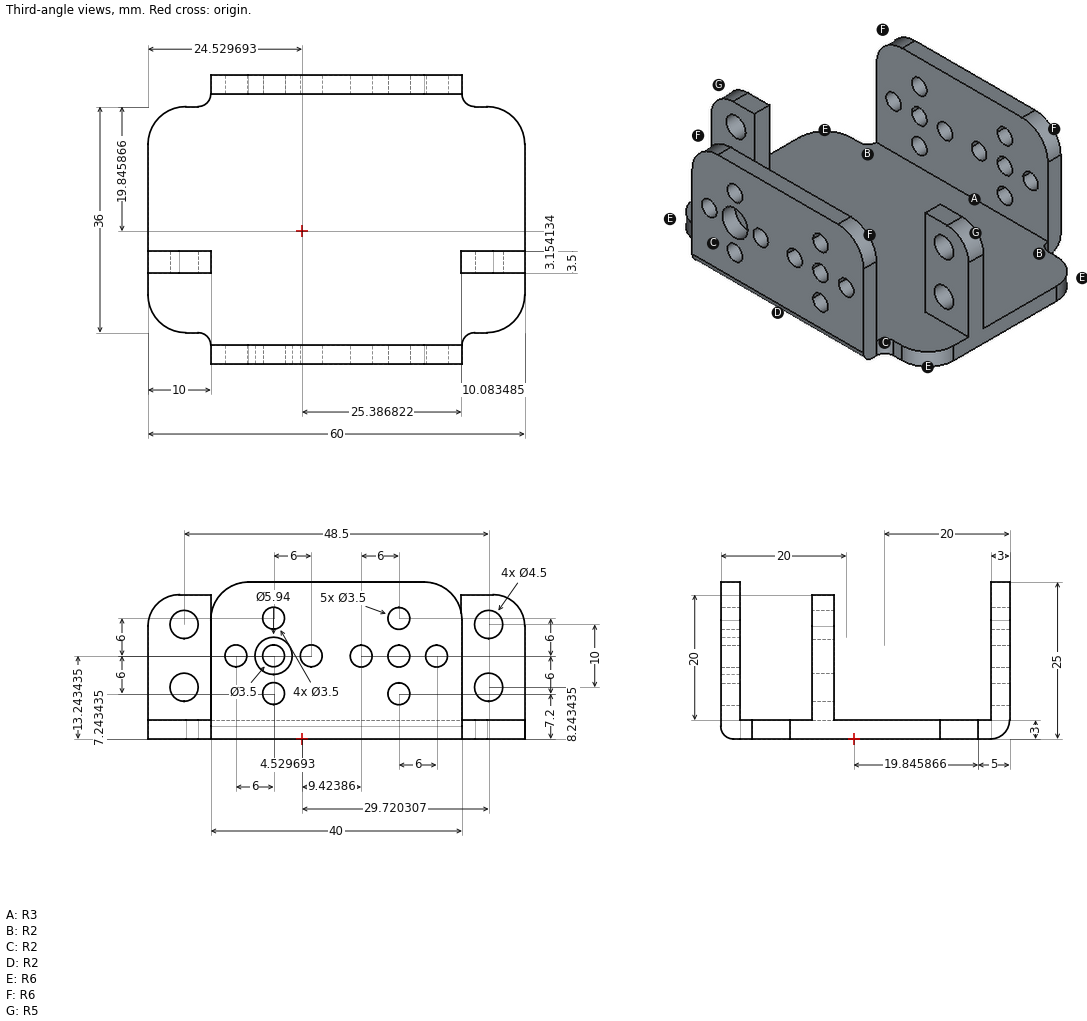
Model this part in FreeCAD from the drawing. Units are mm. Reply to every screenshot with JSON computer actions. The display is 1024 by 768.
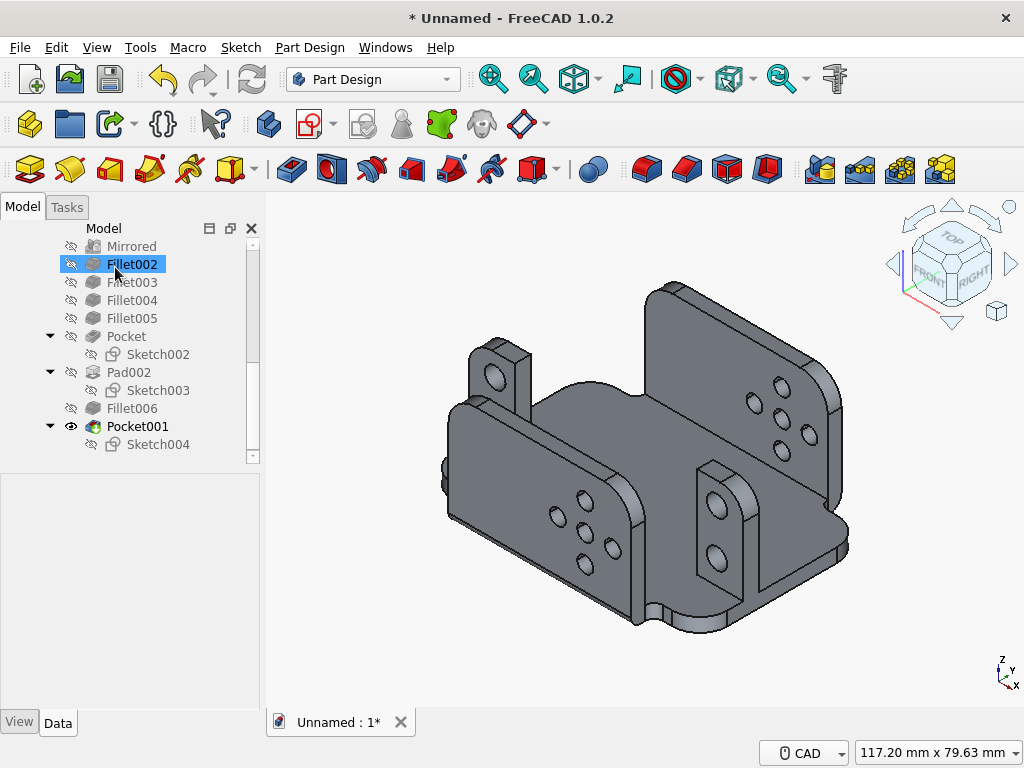
{"action": "left_click", "coordinate": [488, 474]}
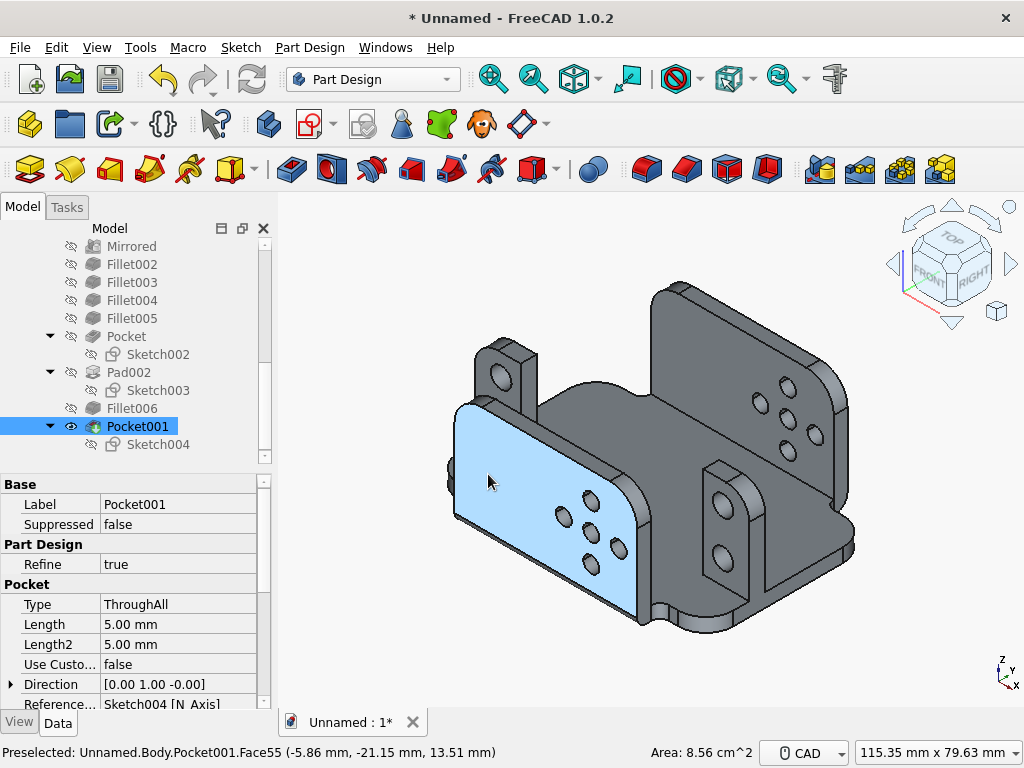
{"action": "left_click", "coordinate": [310, 124]}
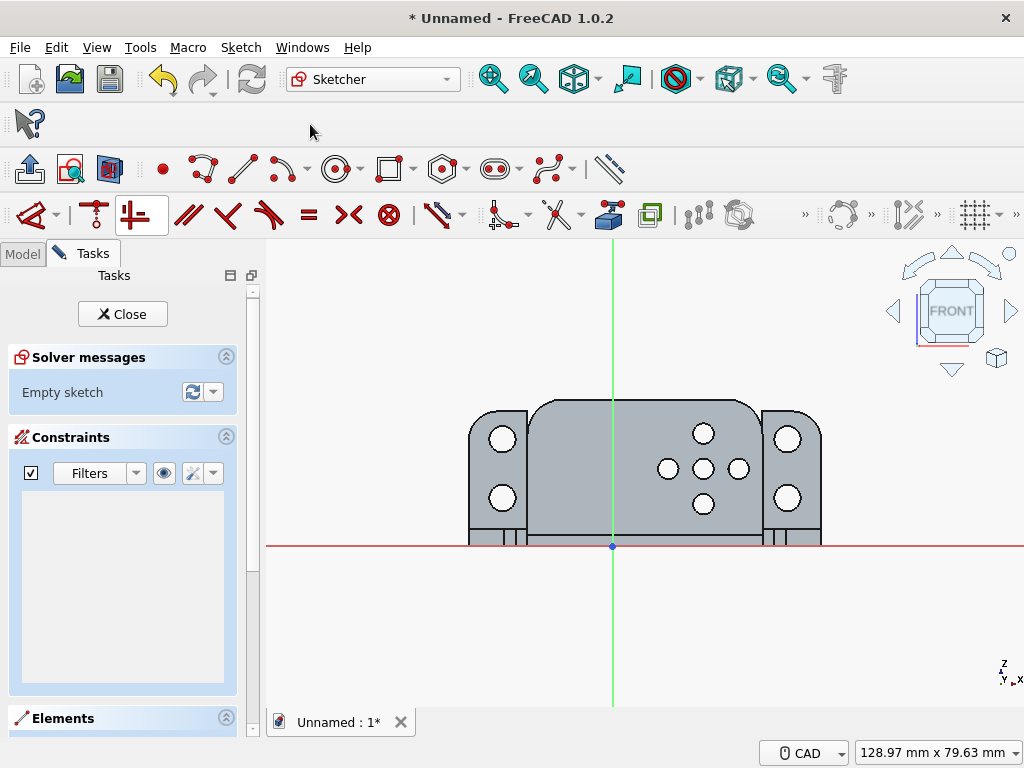
{"action": "scroll", "coordinate": [587, 468], "scroll_direction": "up", "scroll_amount": 11}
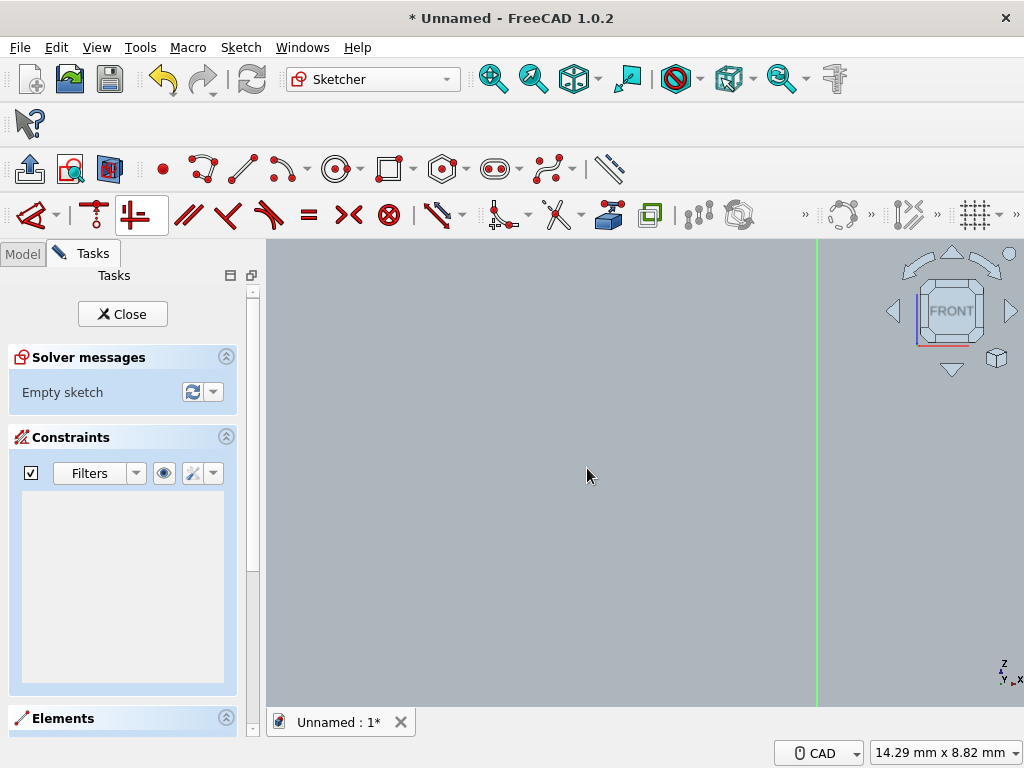
{"action": "left_click", "coordinate": [336, 170]}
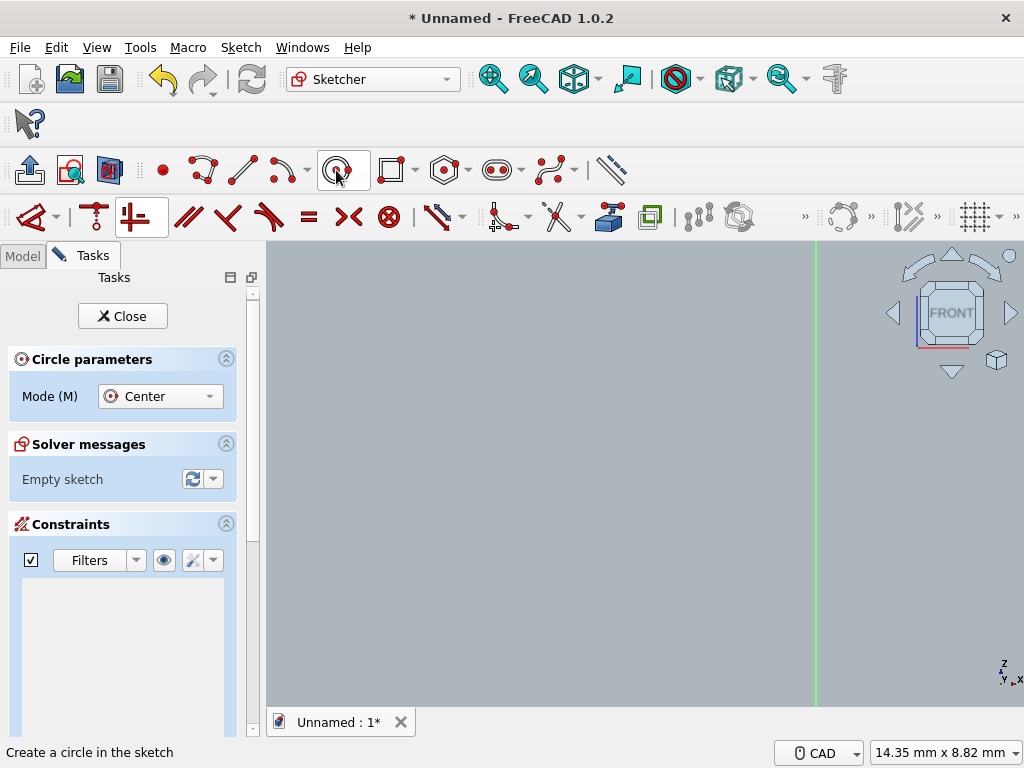
{"action": "left_click", "coordinate": [577, 471]}
{"action": "left_click", "coordinate": [688, 360]}
{"action": "key", "text": "Escape"}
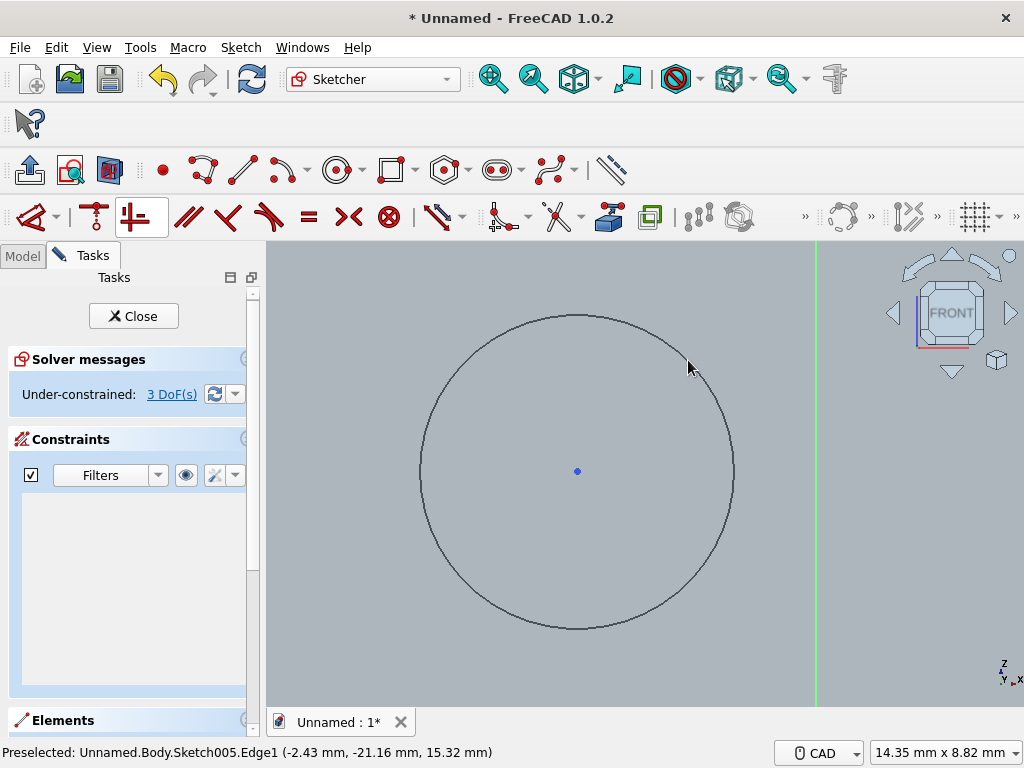
{"action": "left_click", "coordinate": [32, 218]}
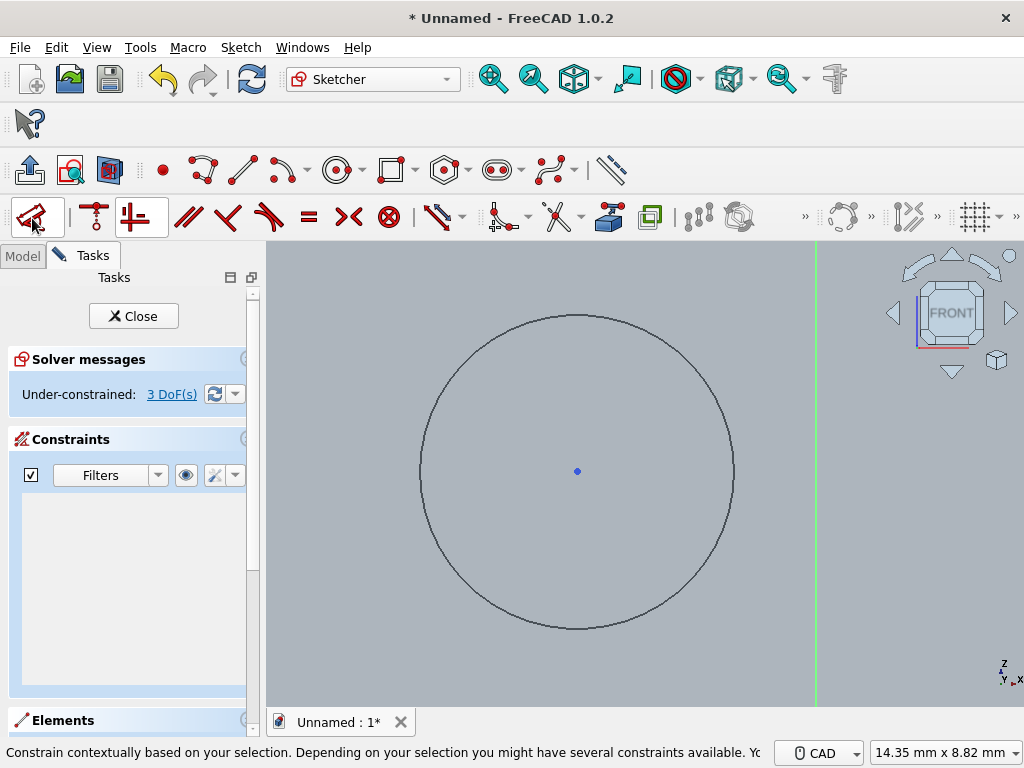
{"action": "left_click", "coordinate": [688, 361]}
{"action": "left_click", "coordinate": [711, 338]}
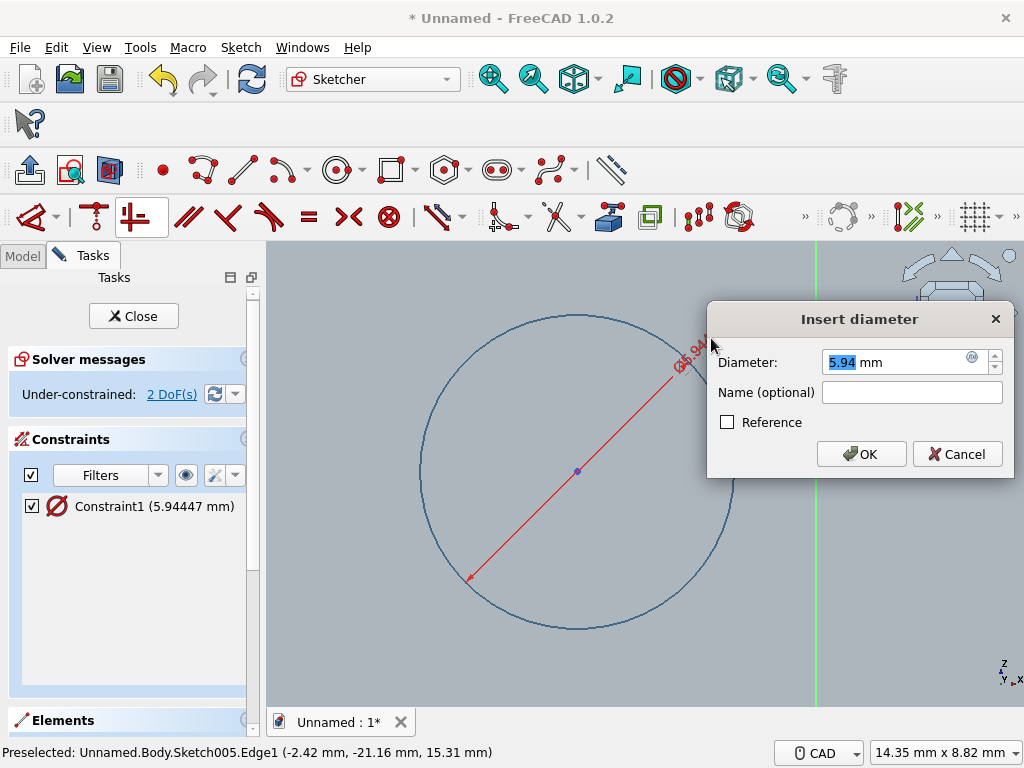
{"action": "type", "text": "5.94"}
{"action": "key", "text": "Return"}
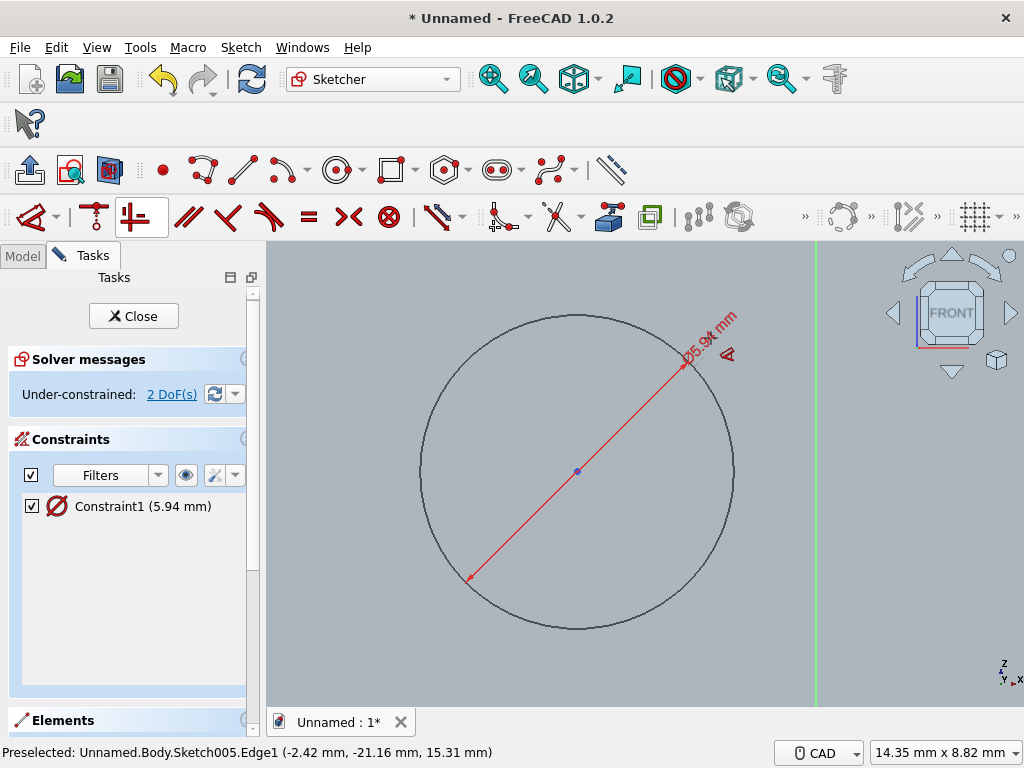
{"action": "left_click", "coordinate": [577, 472]}
{"action": "left_click", "coordinate": [697, 438]}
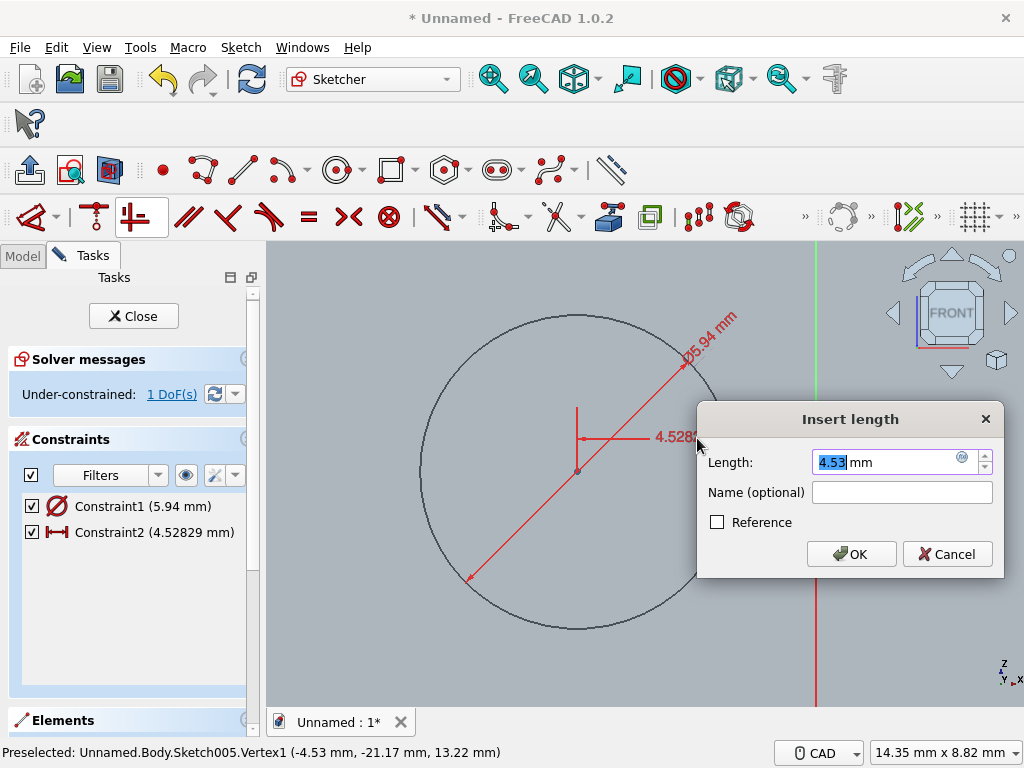
{"action": "type", "text": "4.529693"}
{"action": "key", "text": "Return"}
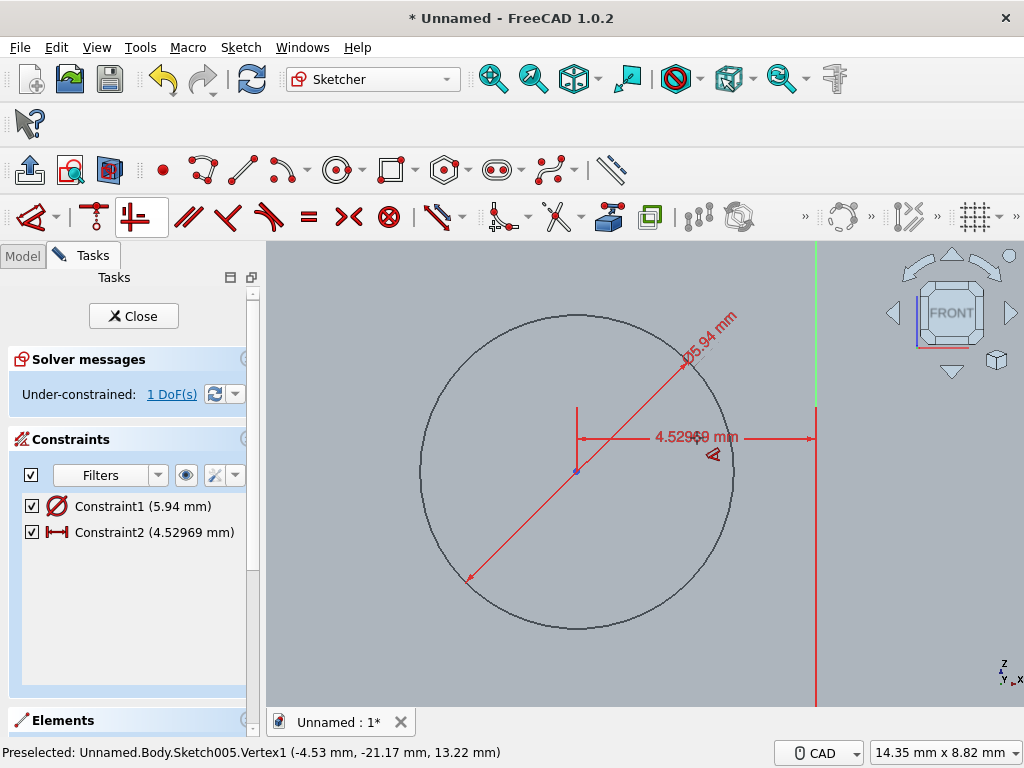
{"action": "left_click", "coordinate": [577, 472]}
{"action": "left_click", "coordinate": [850, 575]}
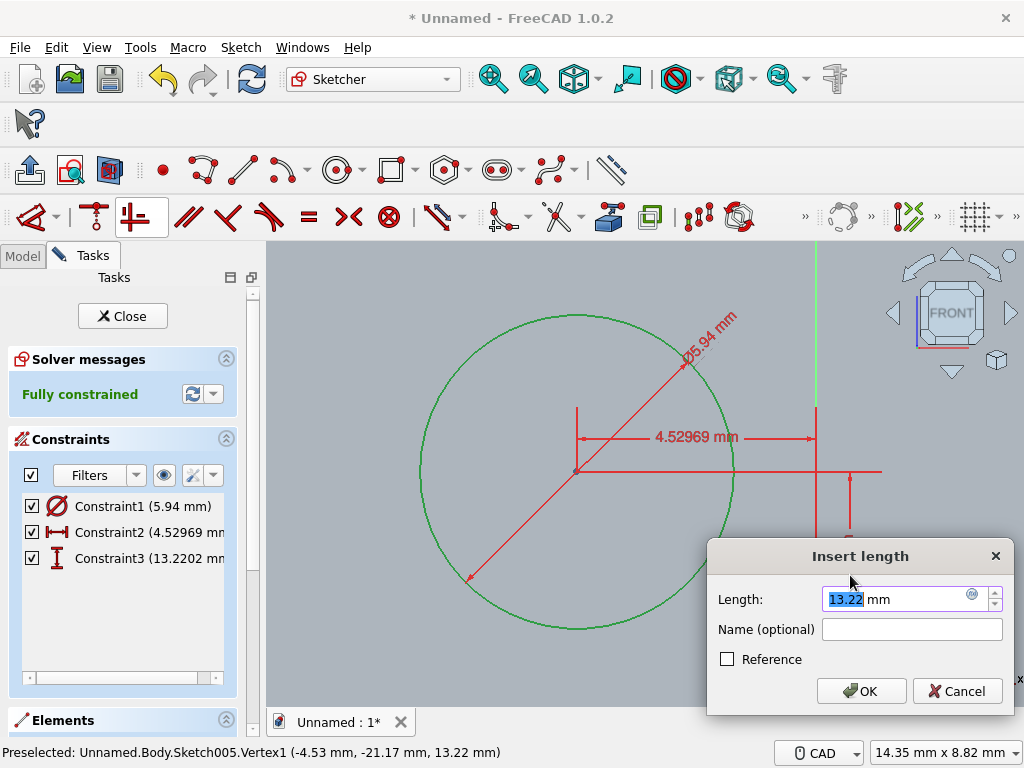
{"action": "type", "text": "13.243435"}
{"action": "key", "text": "Return"}
{"action": "key", "text": "Escape"}